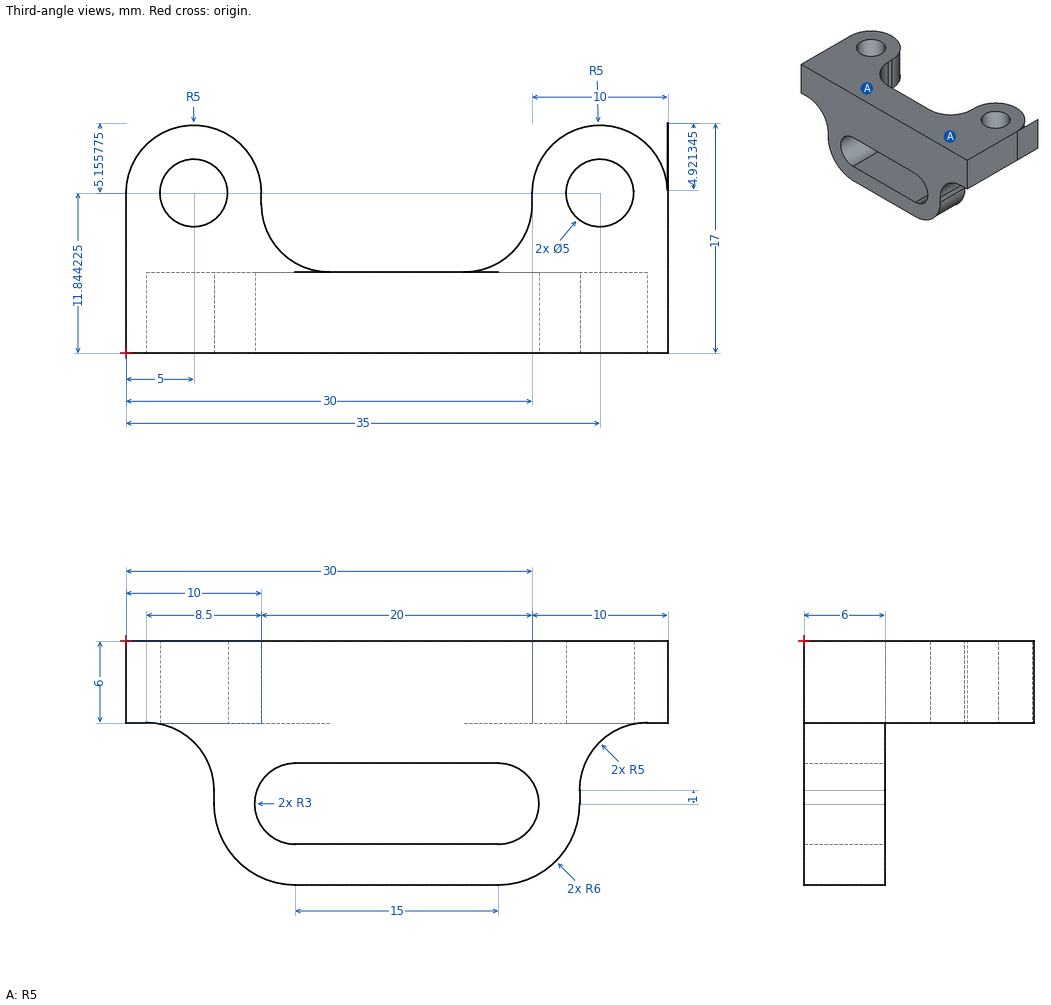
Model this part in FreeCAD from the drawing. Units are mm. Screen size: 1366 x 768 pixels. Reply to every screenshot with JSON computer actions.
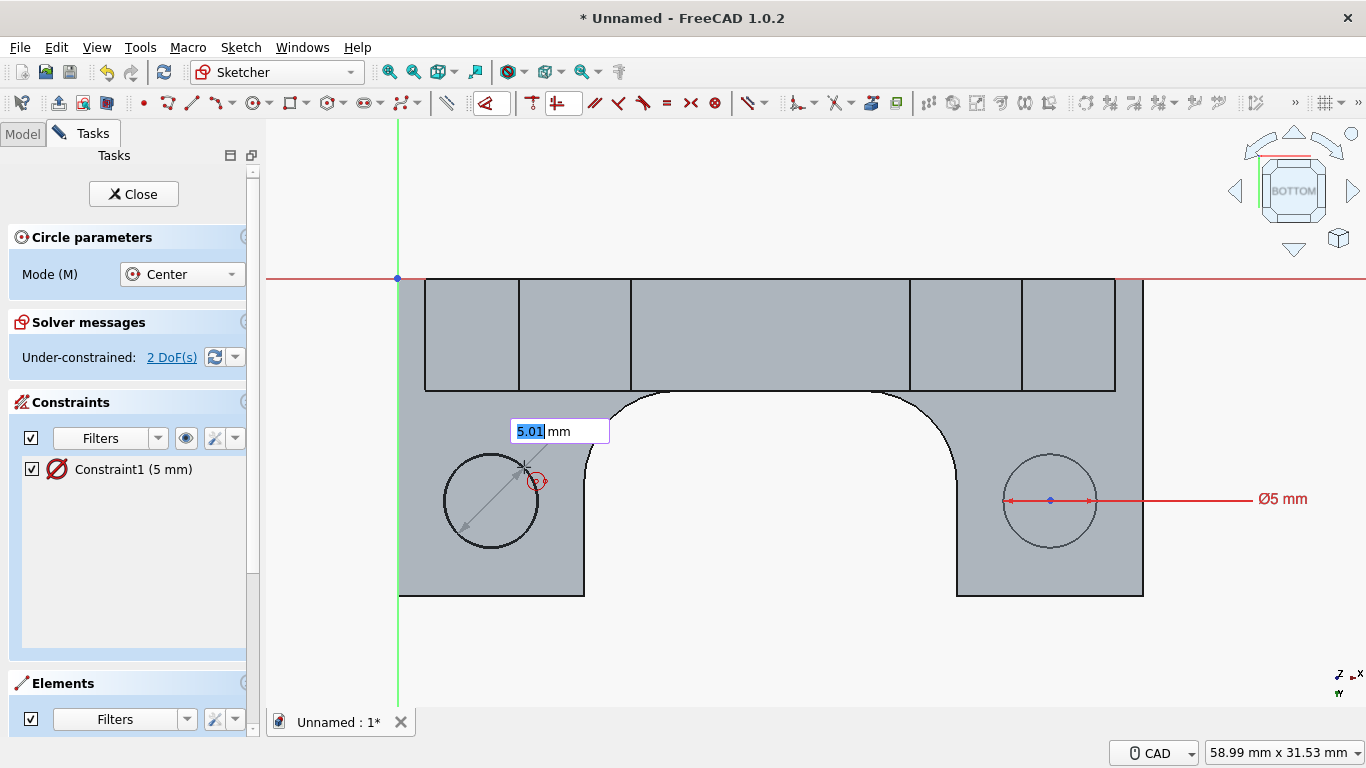
{"action": "type", "text": "5"}
{"action": "key", "text": "Return"}
{"action": "key", "text": "Escape"}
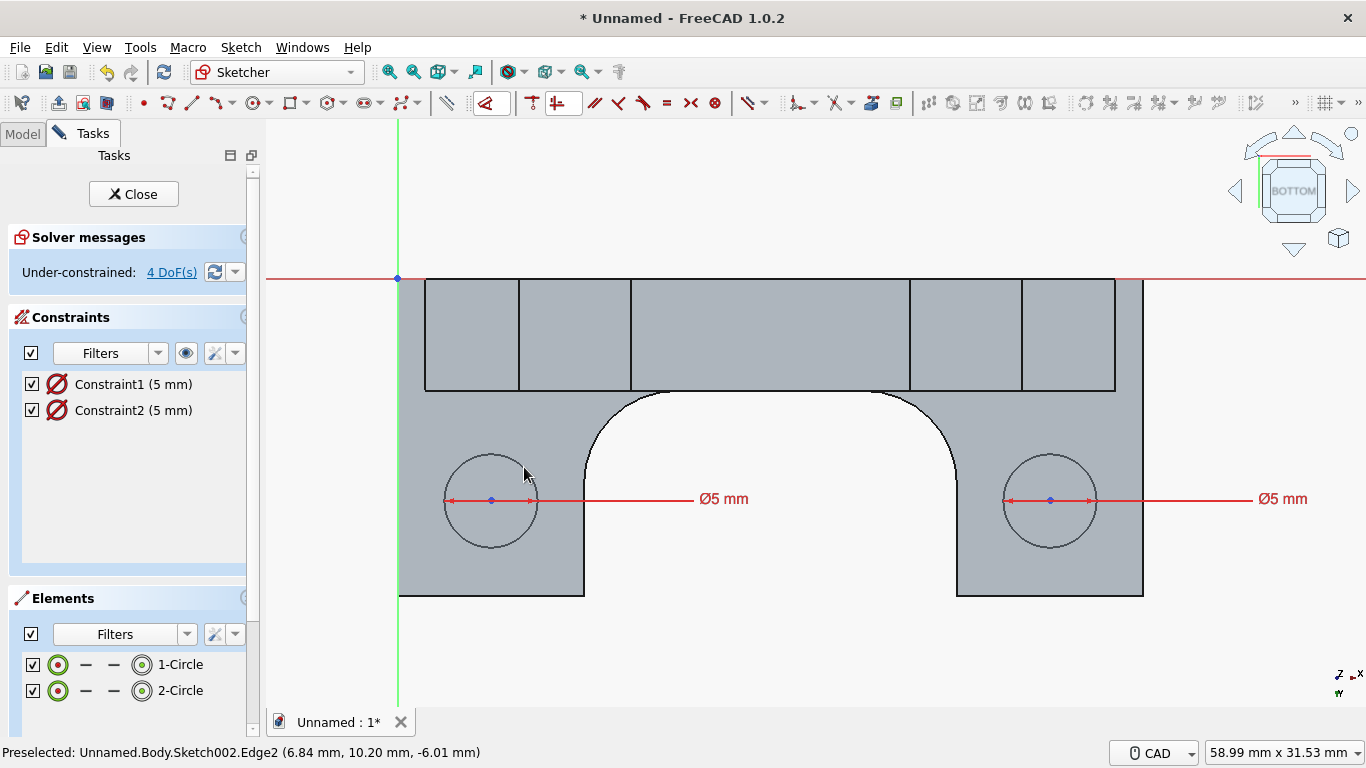
{"action": "left_click", "coordinate": [1050, 501]}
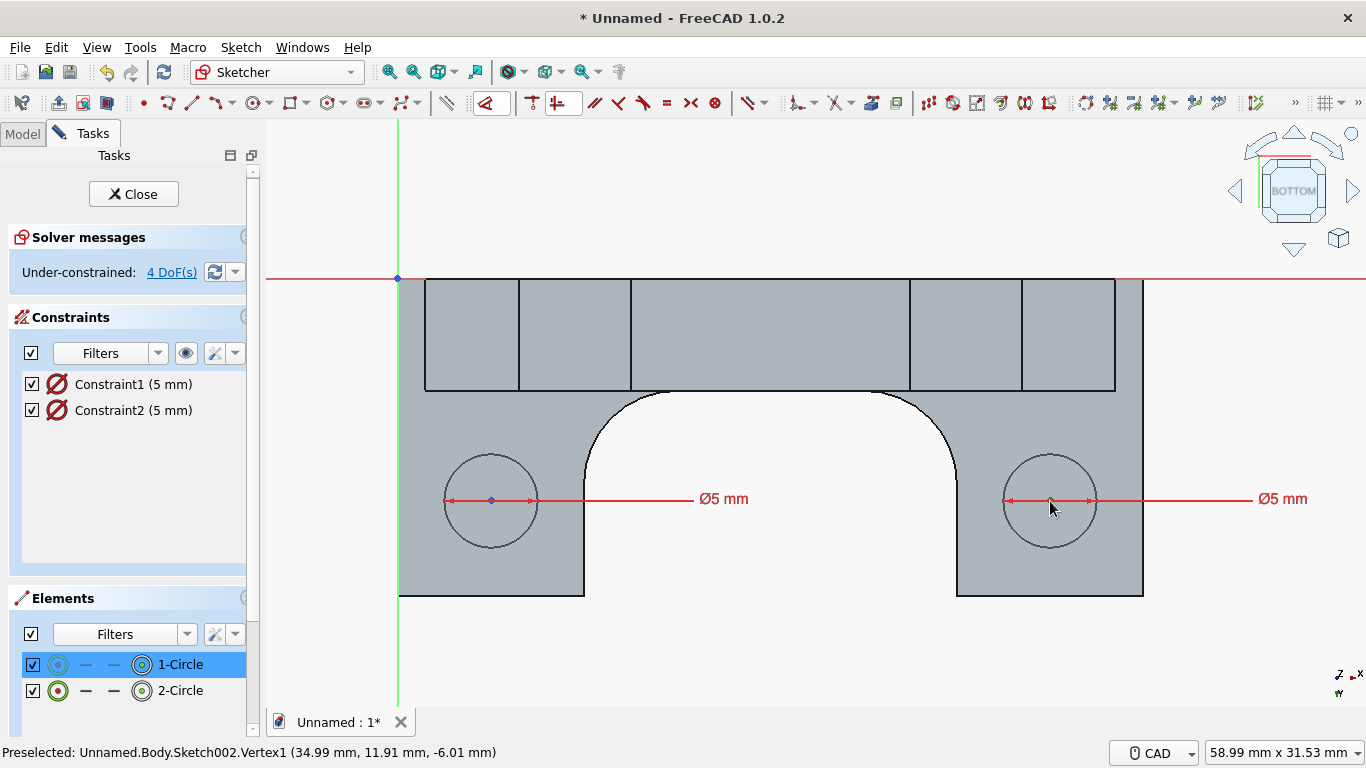
{"action": "left_click", "coordinate": [491, 501]}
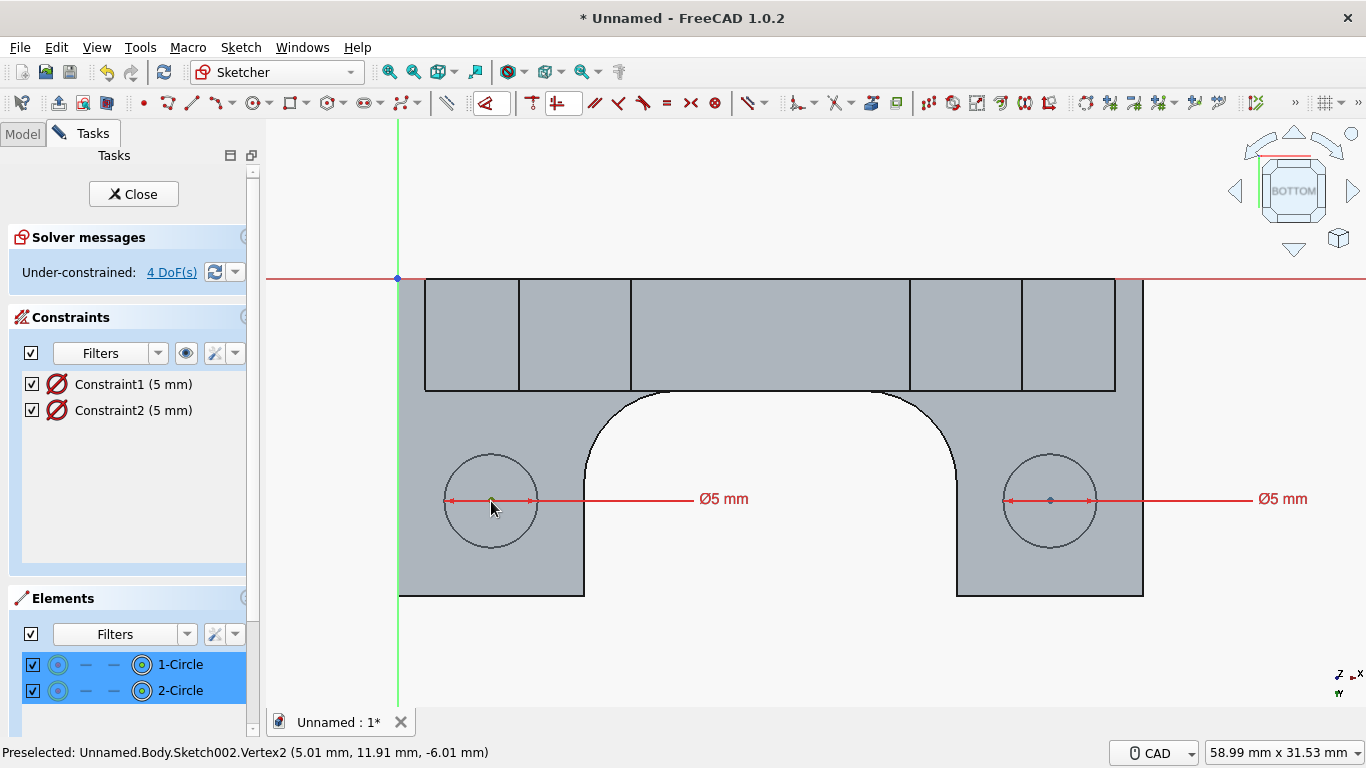
{"action": "key", "text": "h"}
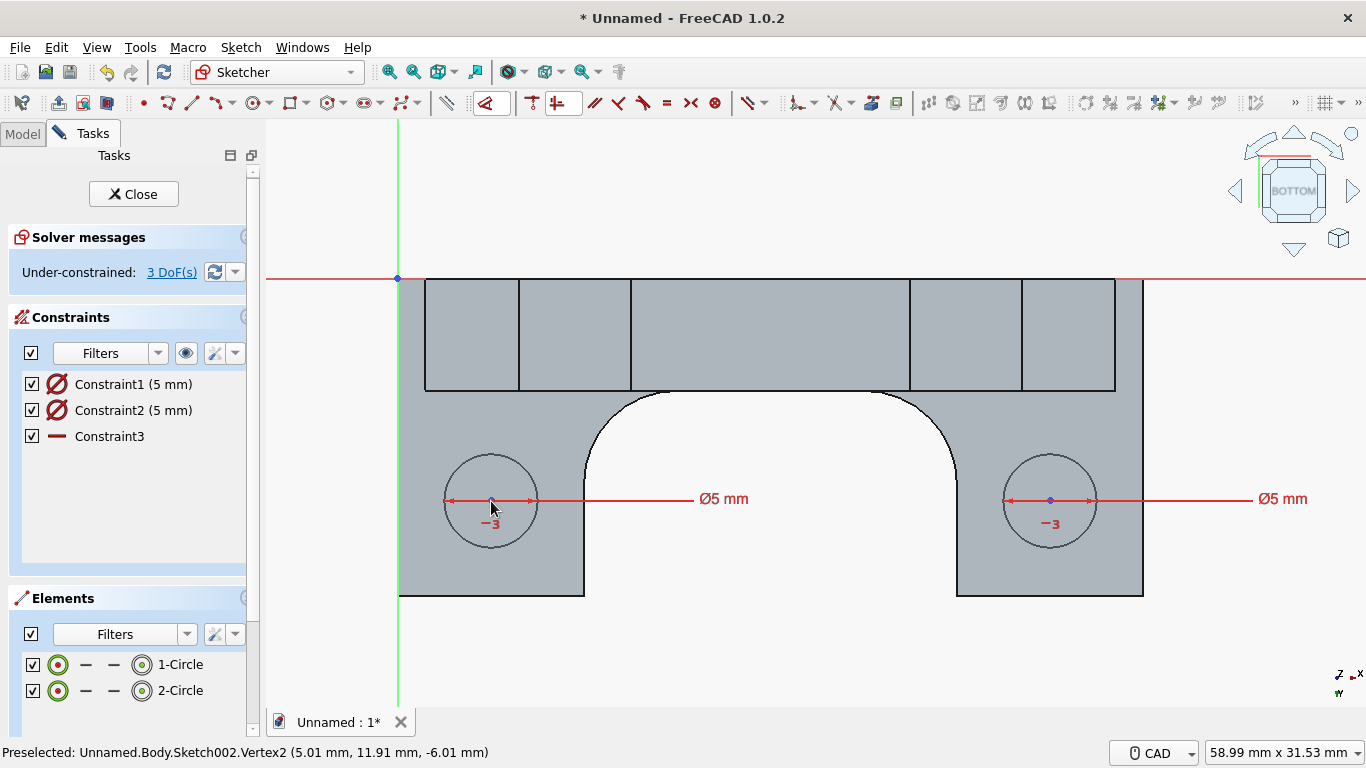
{"action": "left_click", "coordinate": [491, 501]}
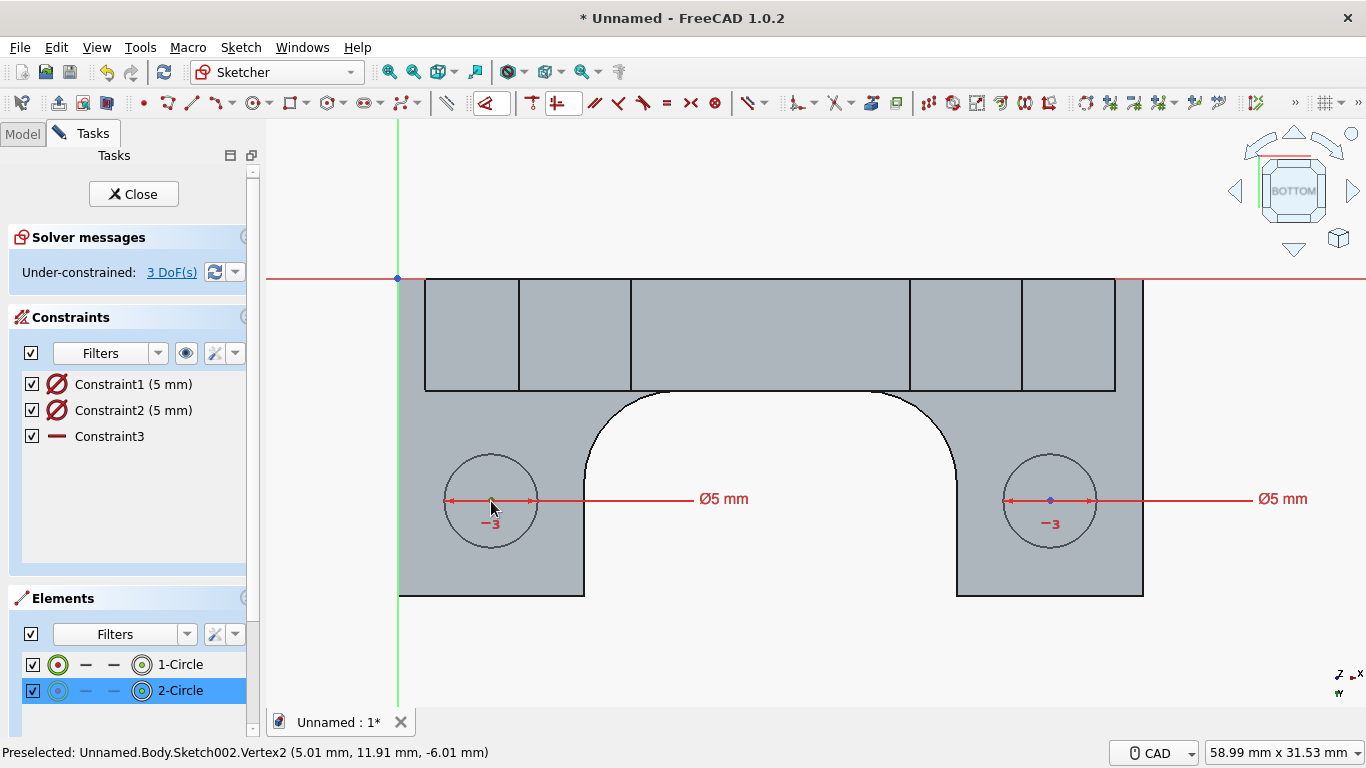
{"action": "key", "text": "l"}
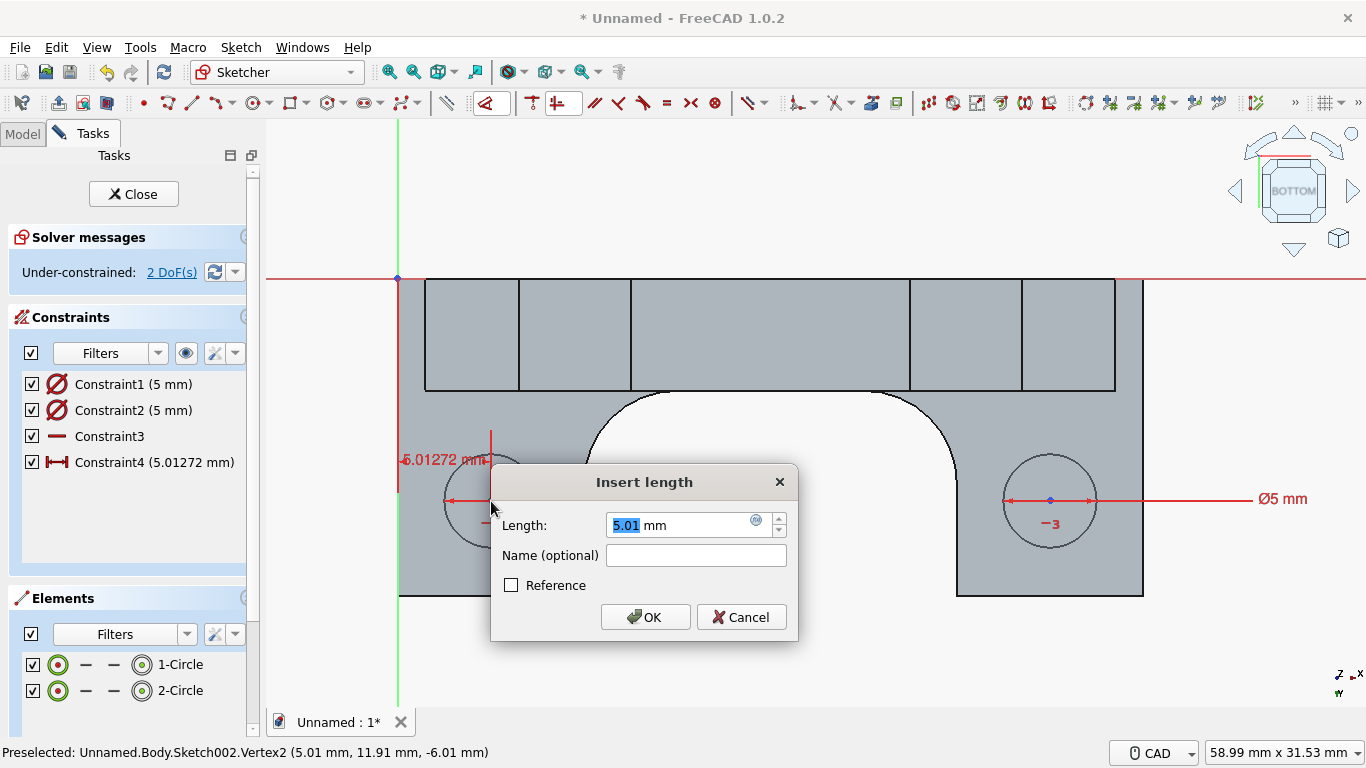
{"action": "type", "text": "5"}
{"action": "key", "text": "Return"}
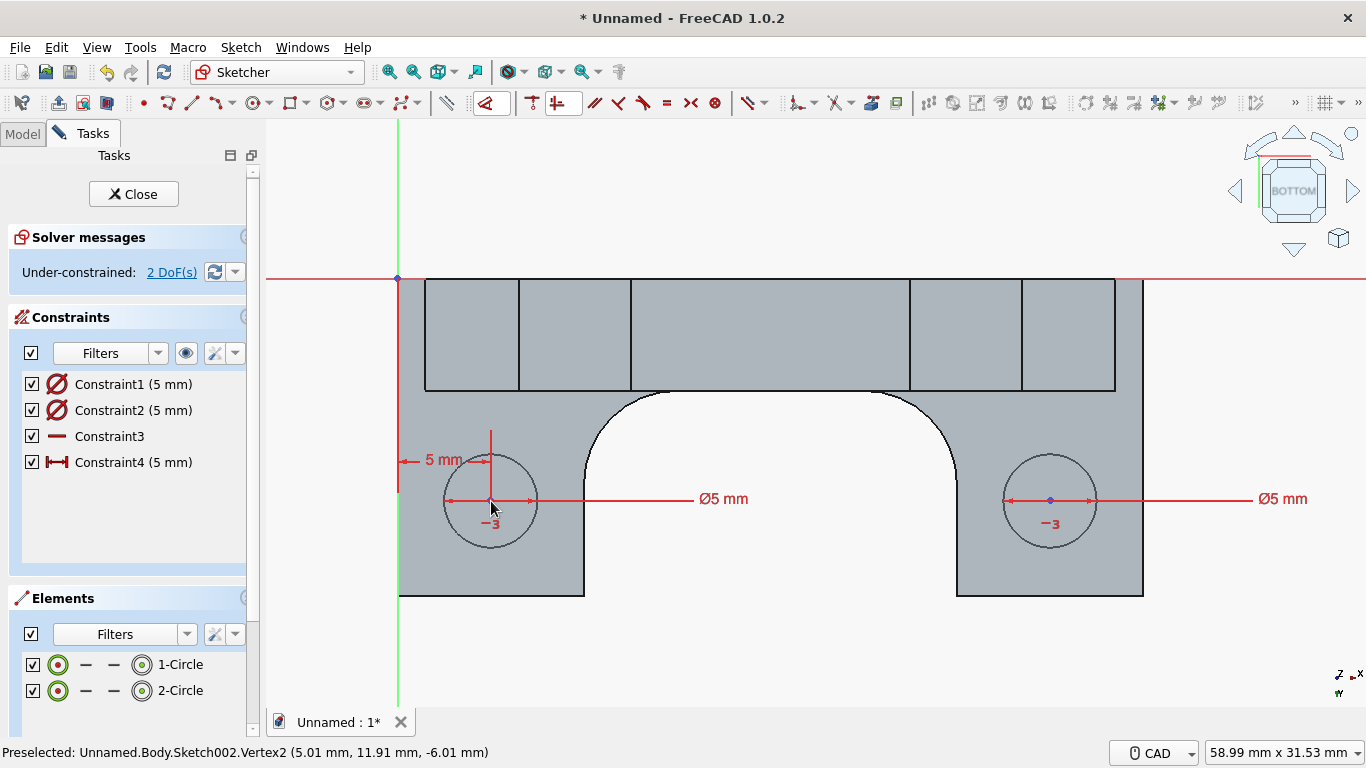
{"action": "left_click", "coordinate": [1050, 501]}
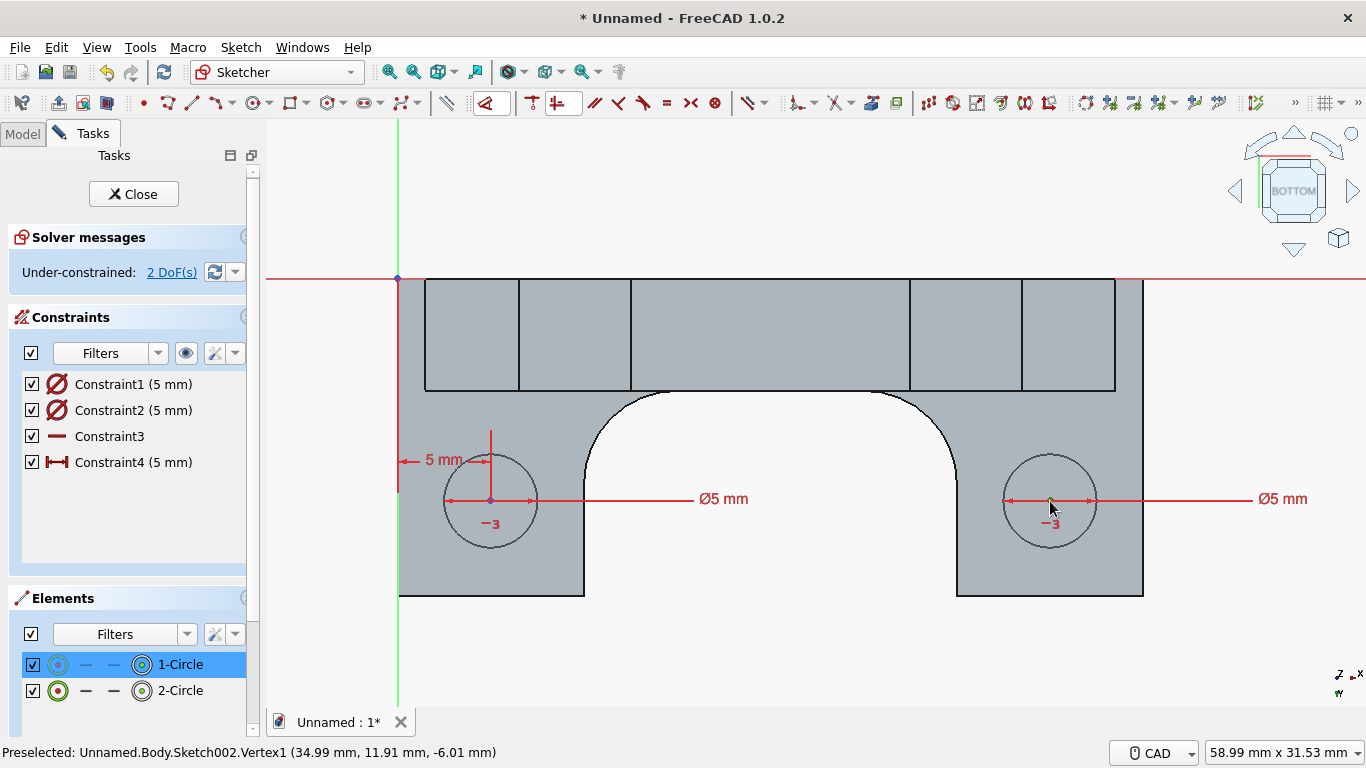
{"action": "left_click", "coordinate": [504, 104]}